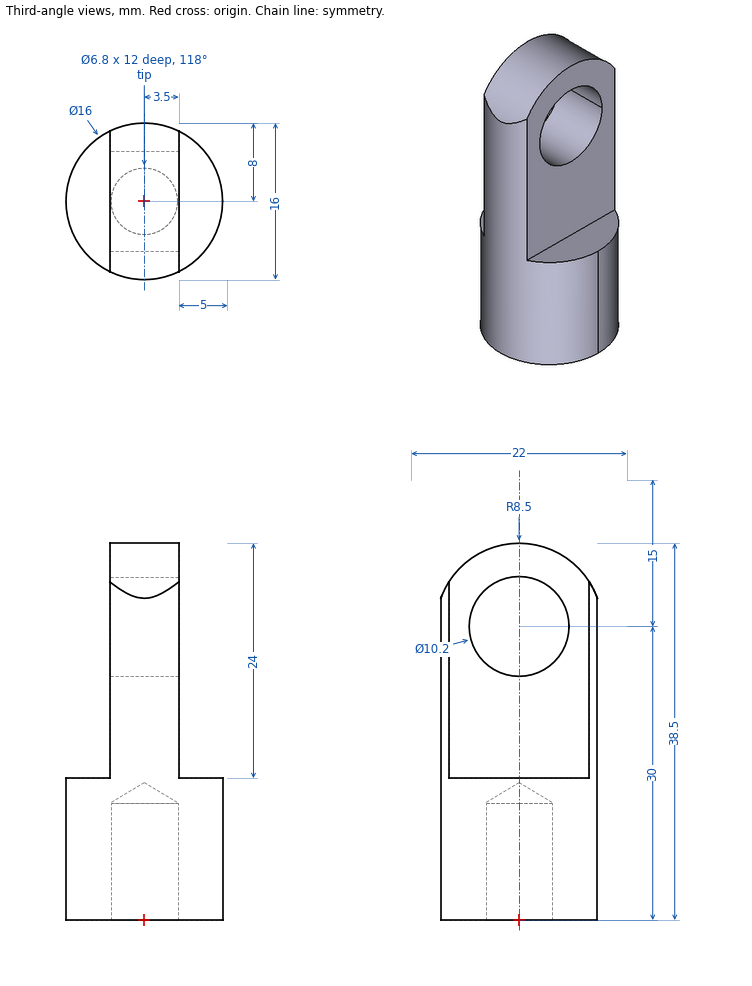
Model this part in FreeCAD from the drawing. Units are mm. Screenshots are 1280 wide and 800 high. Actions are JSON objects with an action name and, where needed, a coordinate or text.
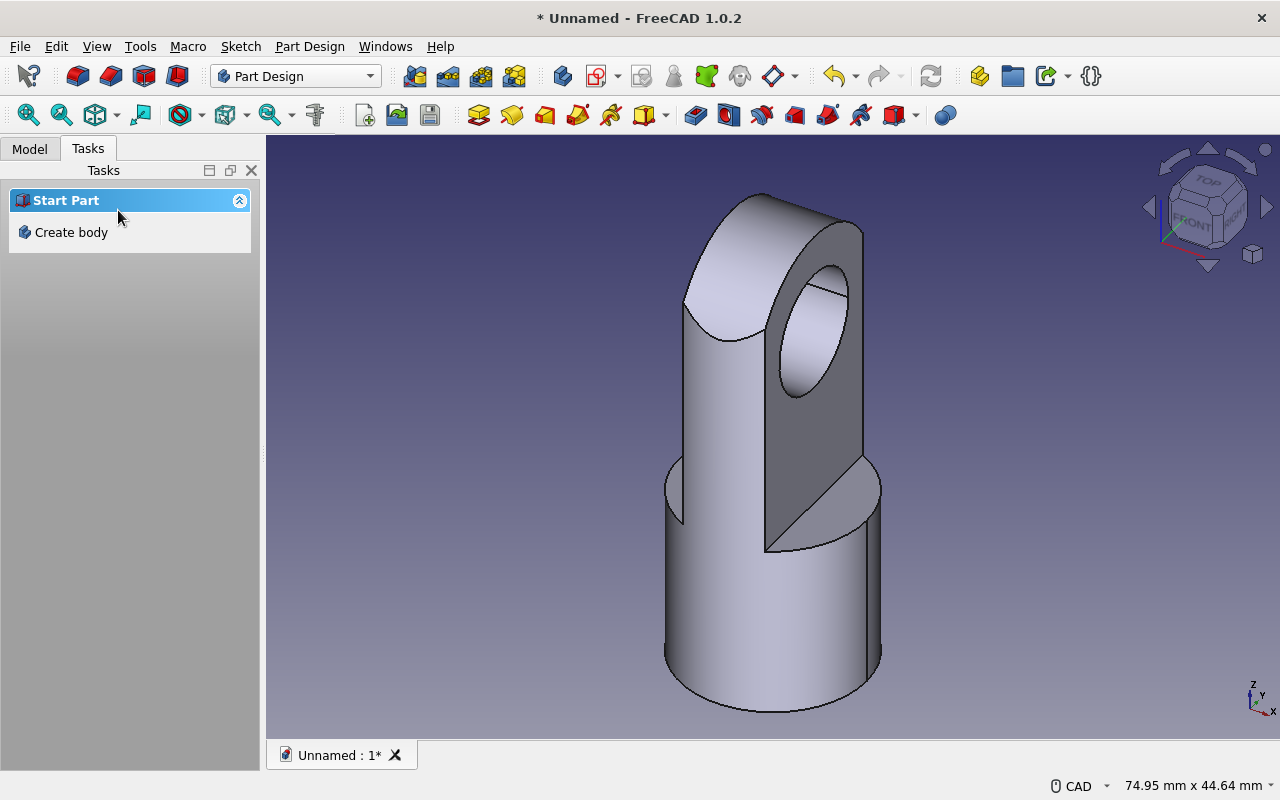
{"action": "left_click", "coordinate": [596, 76]}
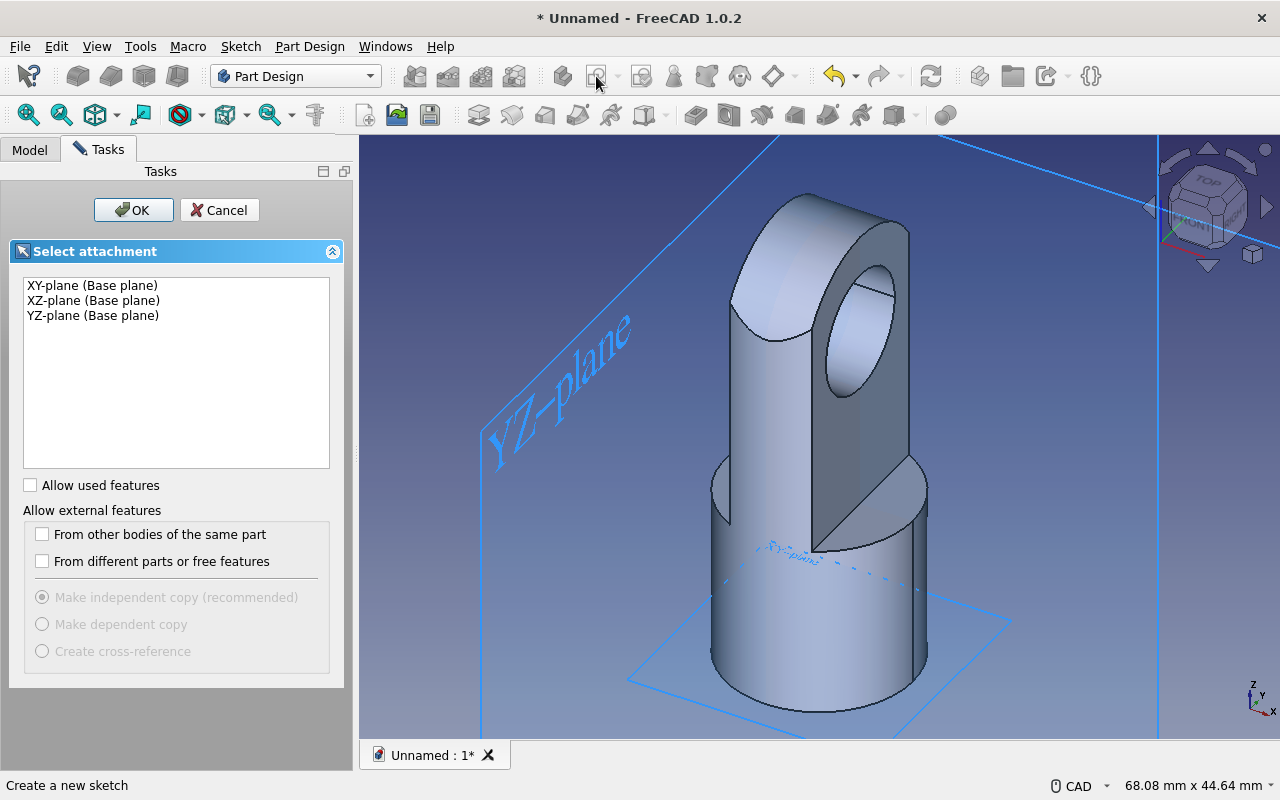
{"action": "left_click", "coordinate": [84, 286]}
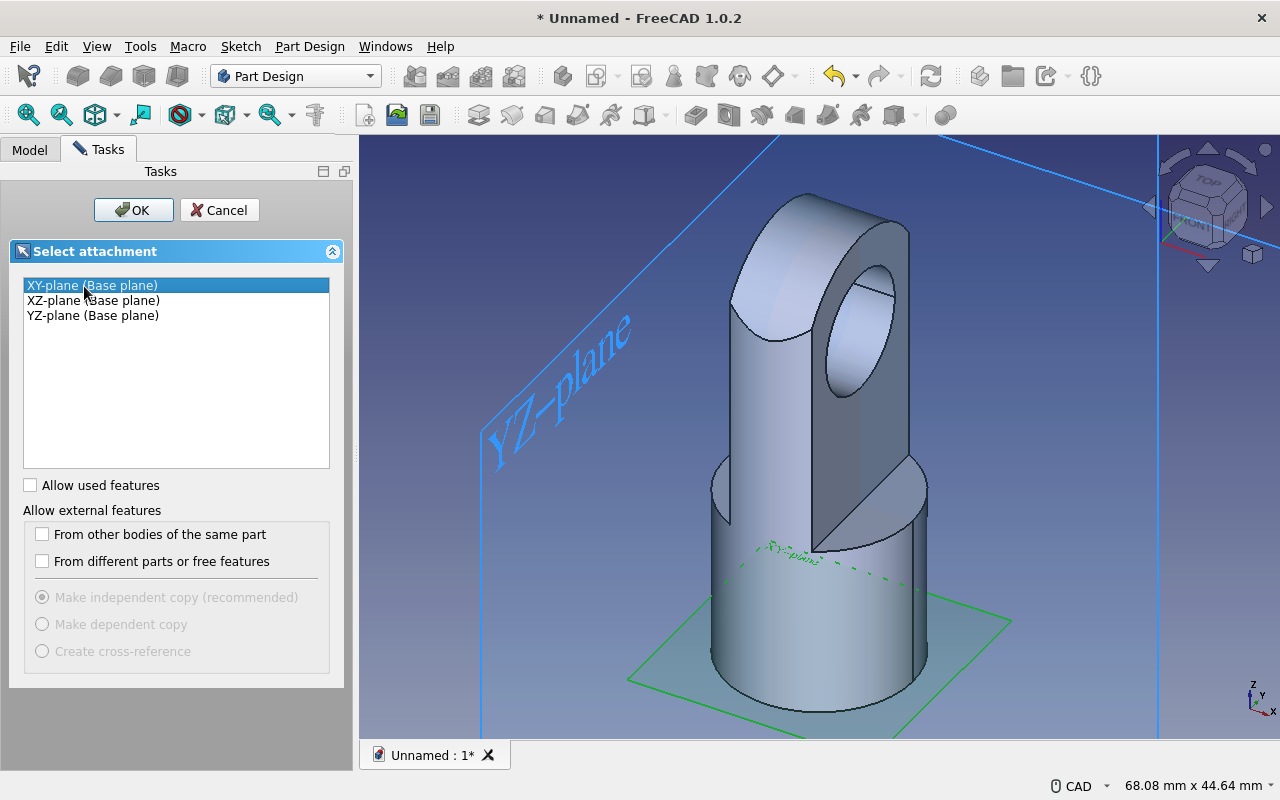
{"action": "left_click", "coordinate": [134, 210]}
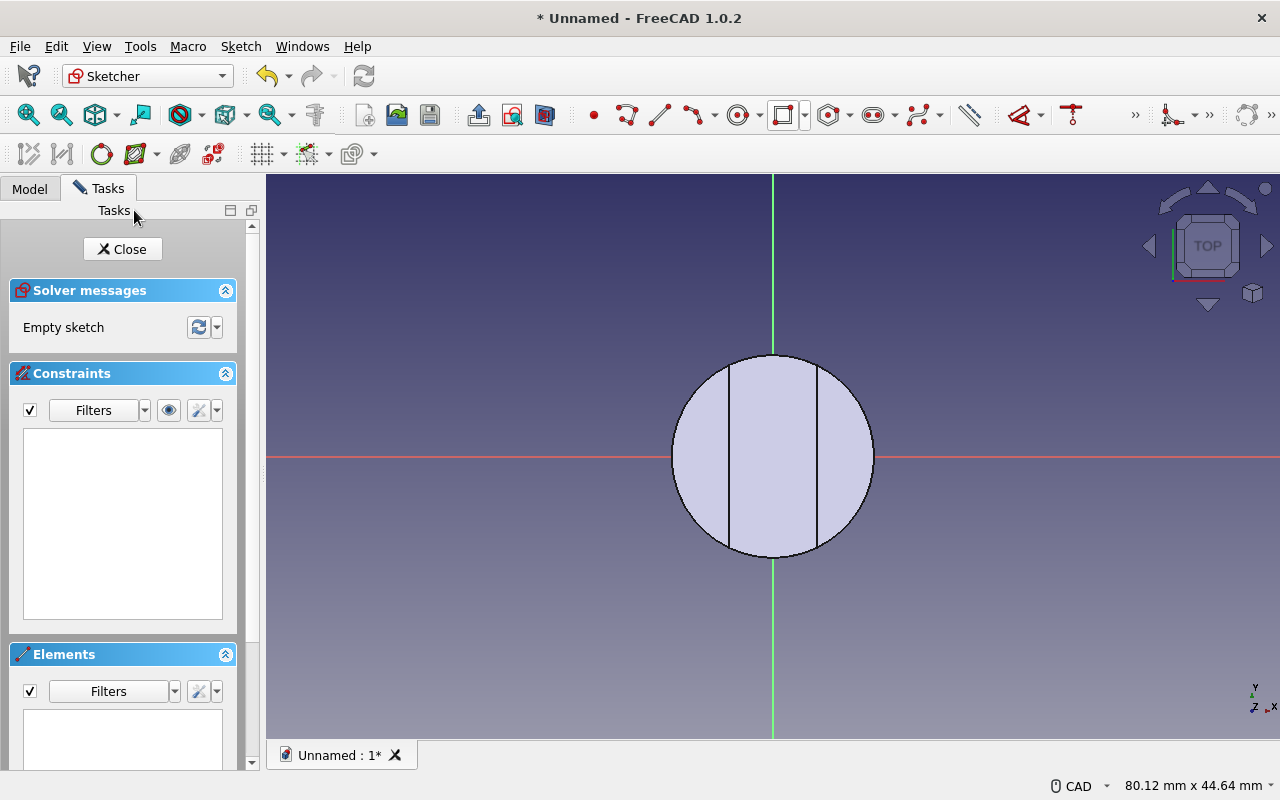
{"action": "key", "text": "q s"}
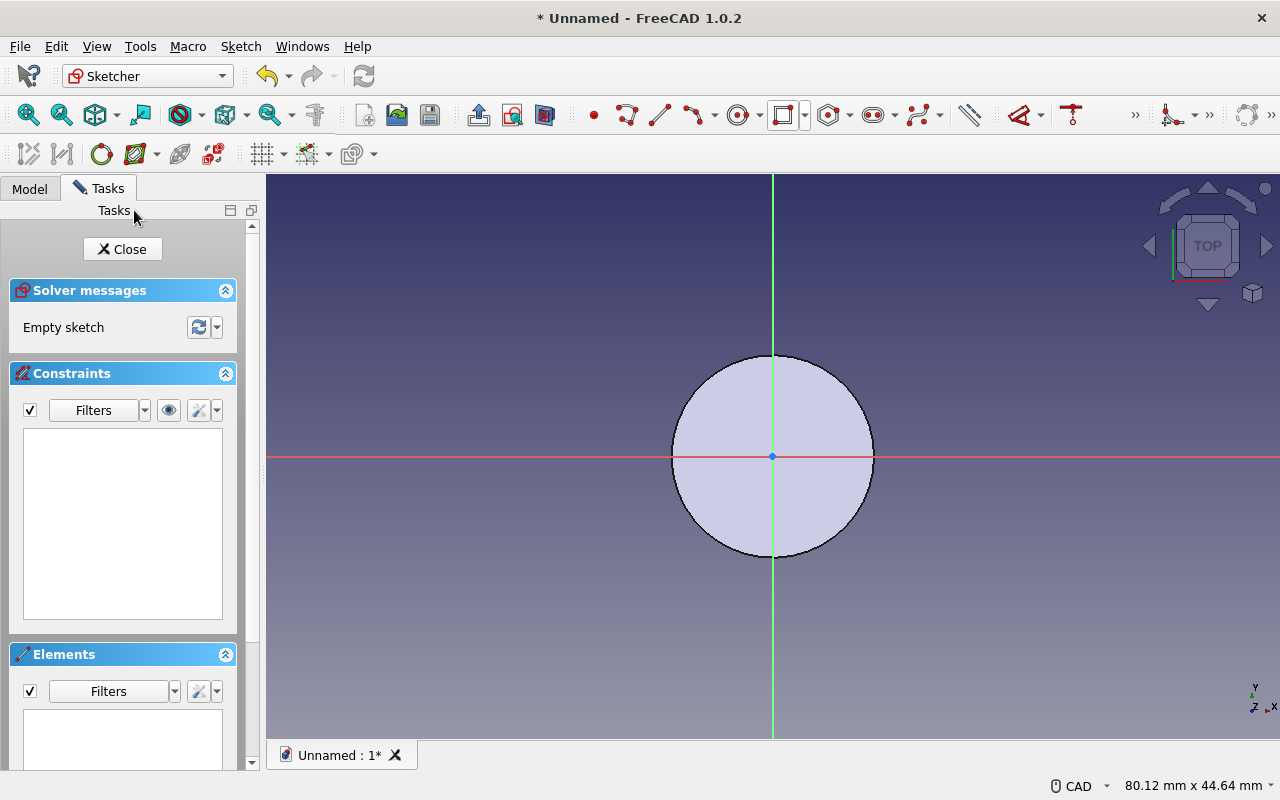
{"action": "scroll", "coordinate": [795, 457], "scroll_direction": "up", "scroll_amount": 7}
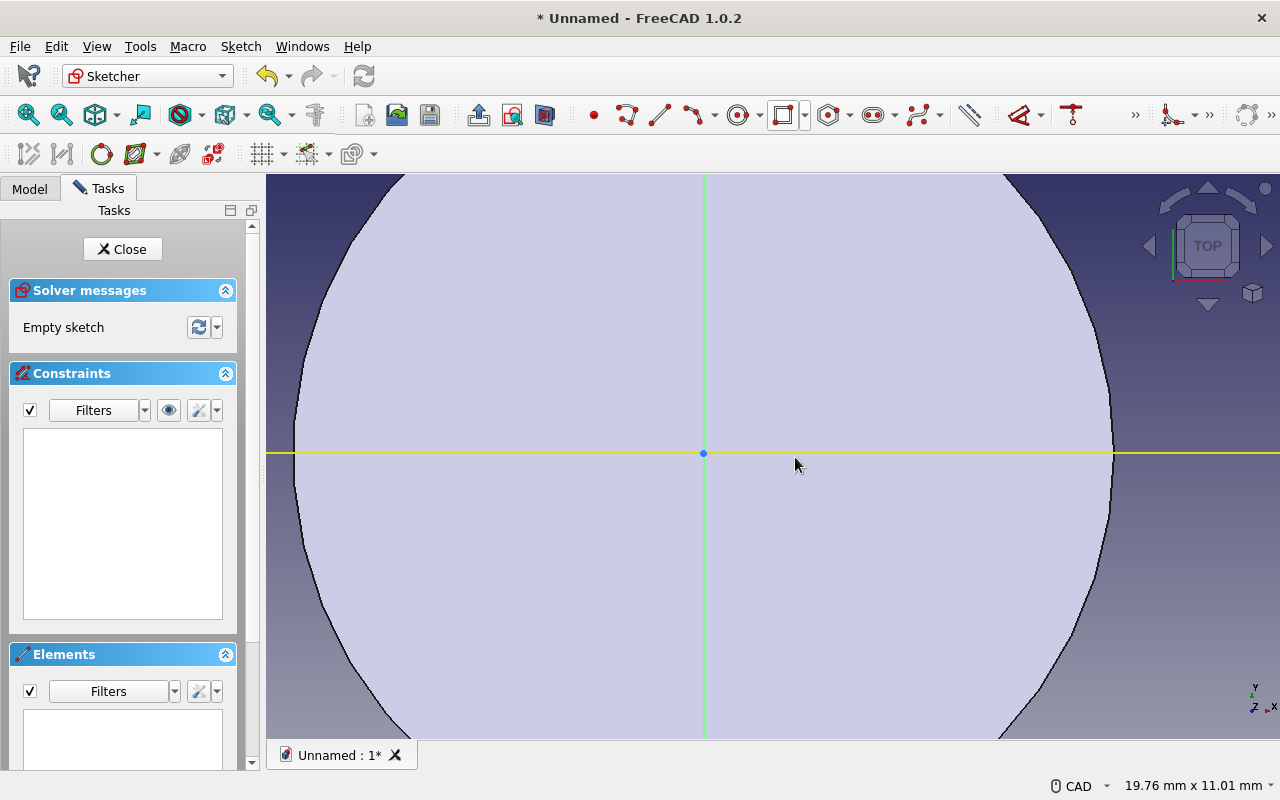
{"action": "left_click", "coordinate": [738, 116]}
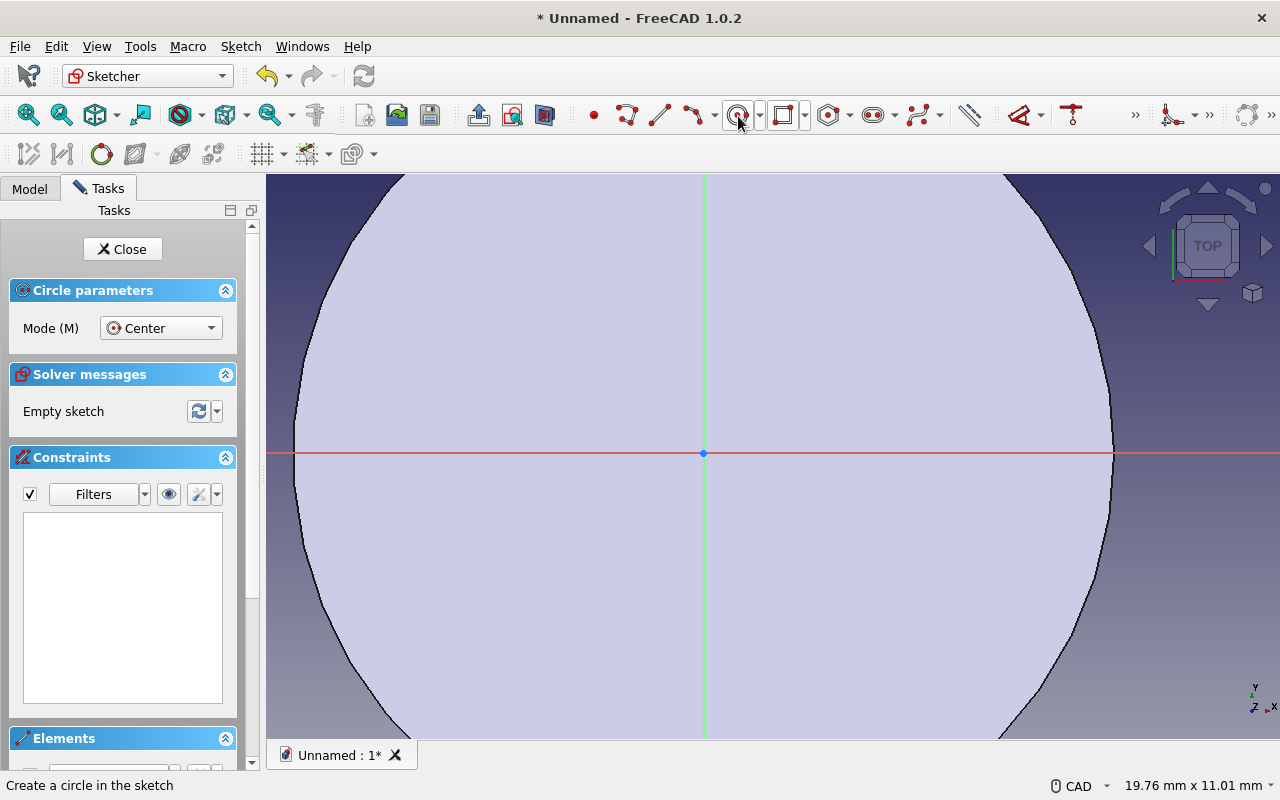
{"action": "left_click", "coordinate": [704, 453]}
{"action": "left_click", "coordinate": [827, 330]}
{"action": "key", "text": "Escape"}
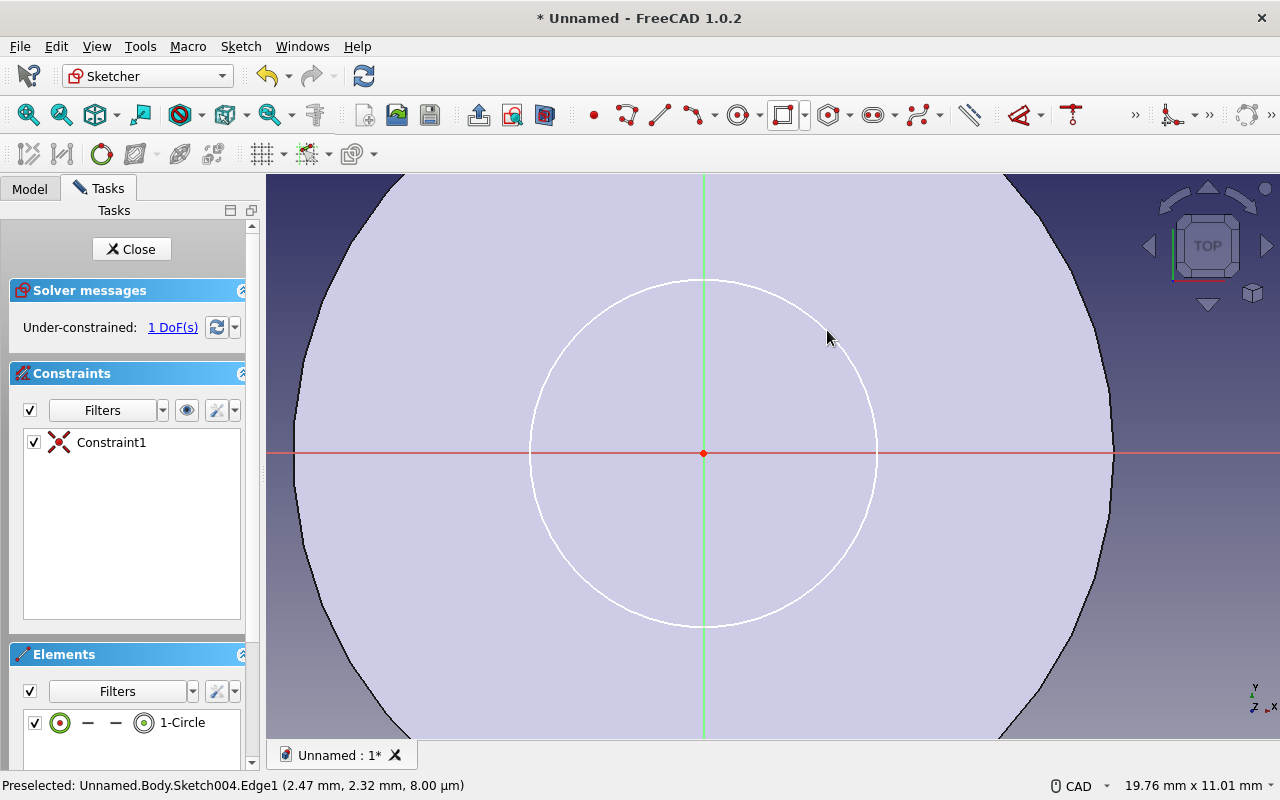
{"action": "key", "text": "d"}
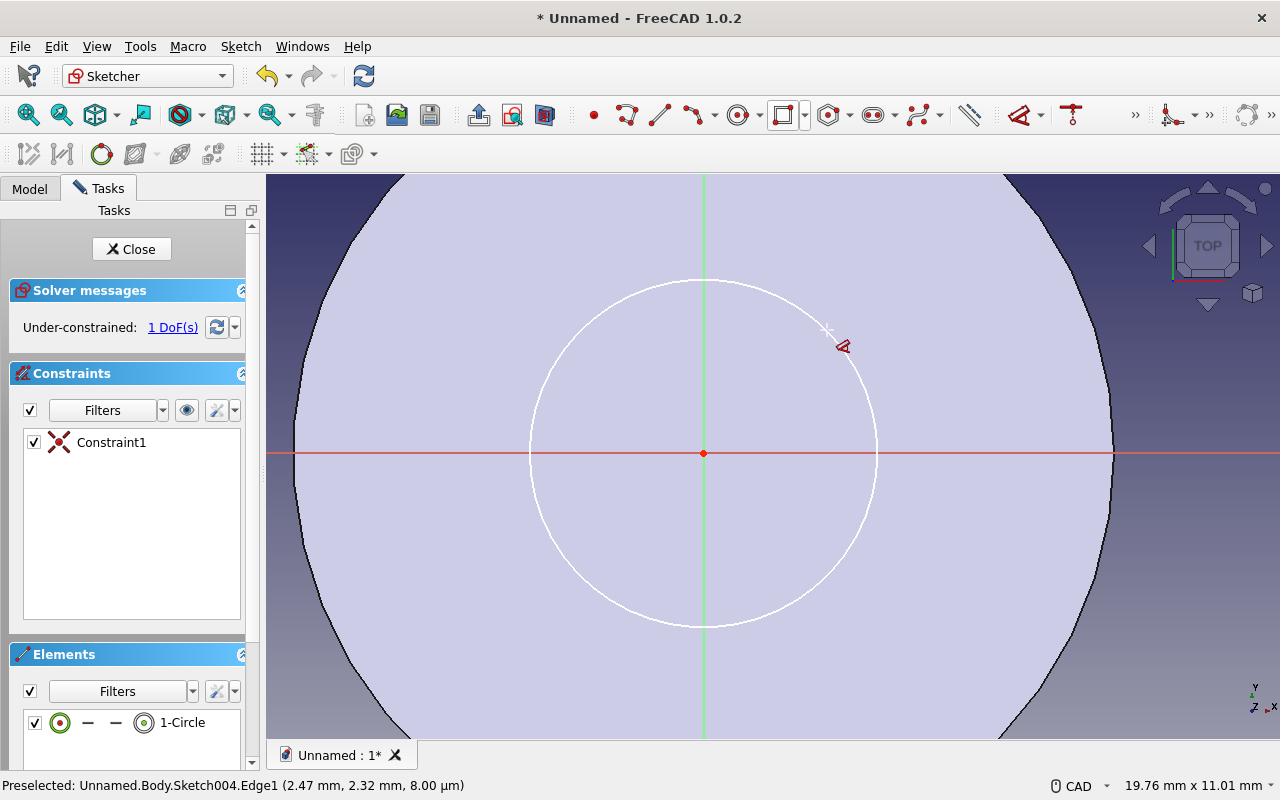
{"action": "left_click", "coordinate": [826, 330]}
{"action": "left_click", "coordinate": [849, 307]}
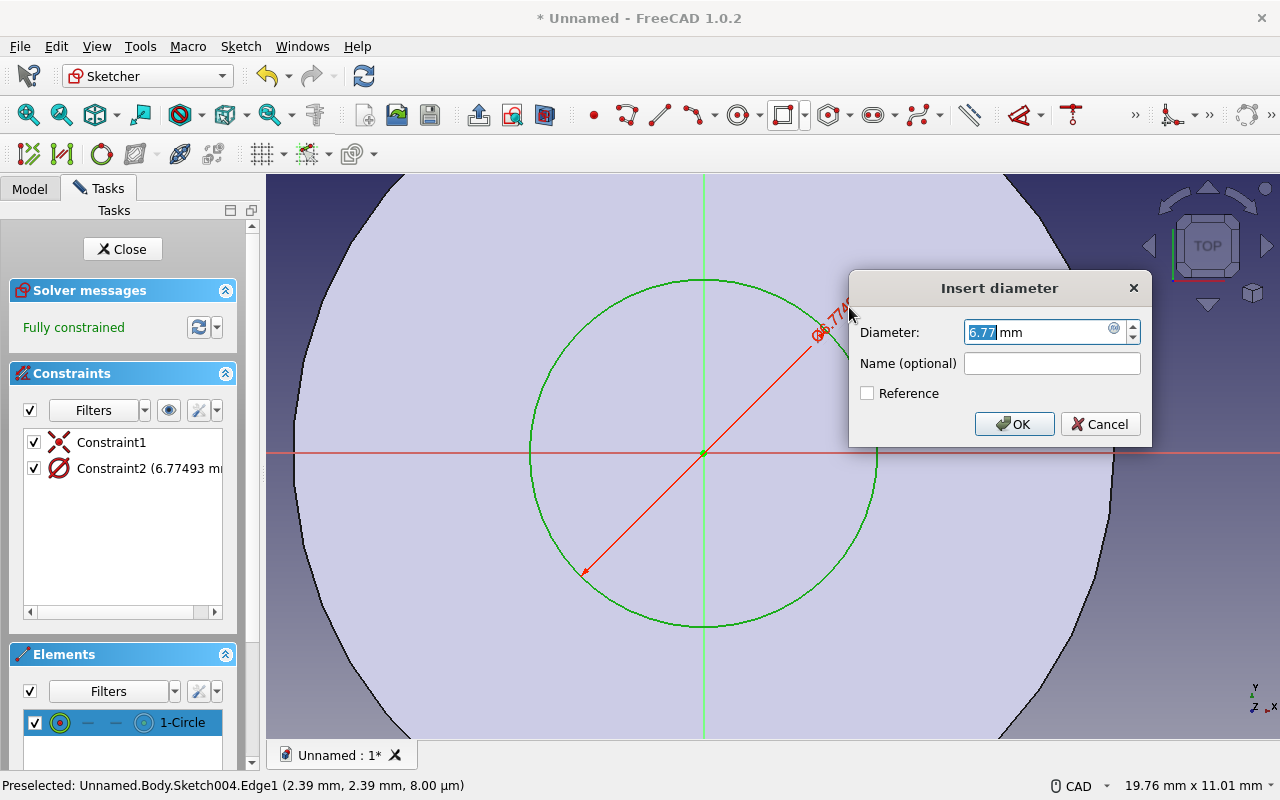
{"action": "type", "text": "6.8"}
{"action": "key", "text": "Return"}
{"action": "key", "text": "Escape"}